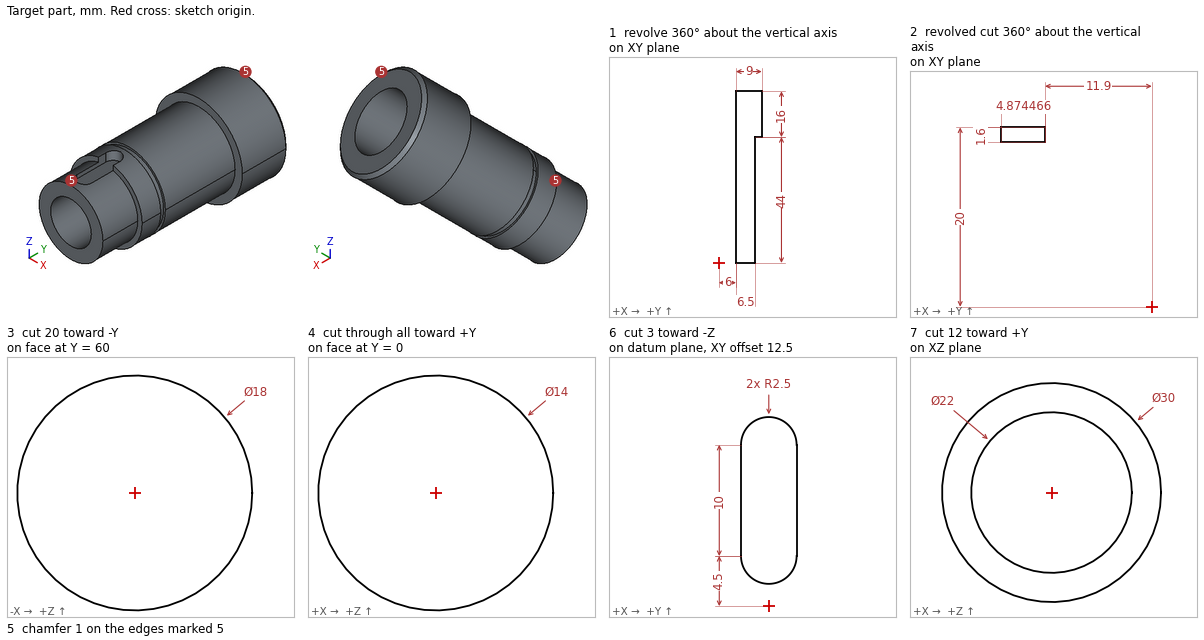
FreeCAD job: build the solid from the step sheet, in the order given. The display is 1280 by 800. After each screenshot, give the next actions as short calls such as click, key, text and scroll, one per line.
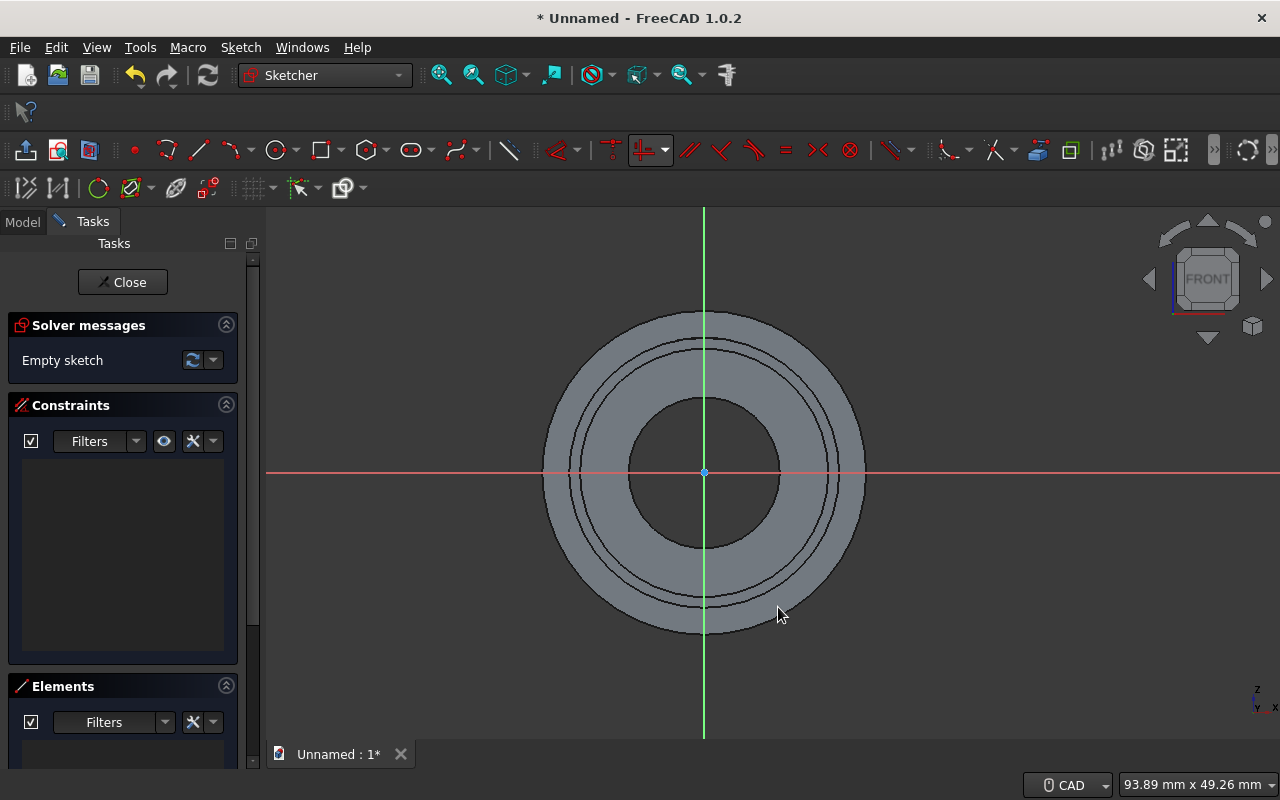
click(276, 150)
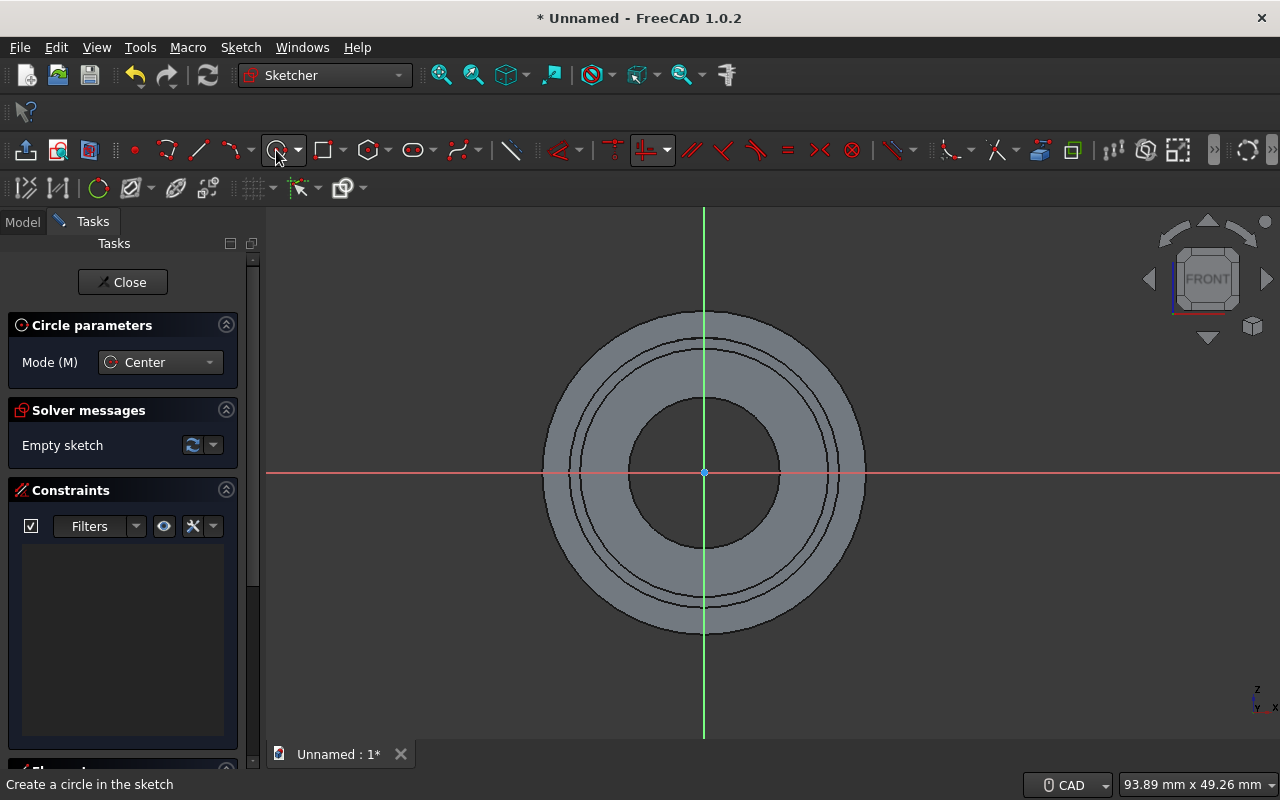
click(704, 473)
move(819, 358)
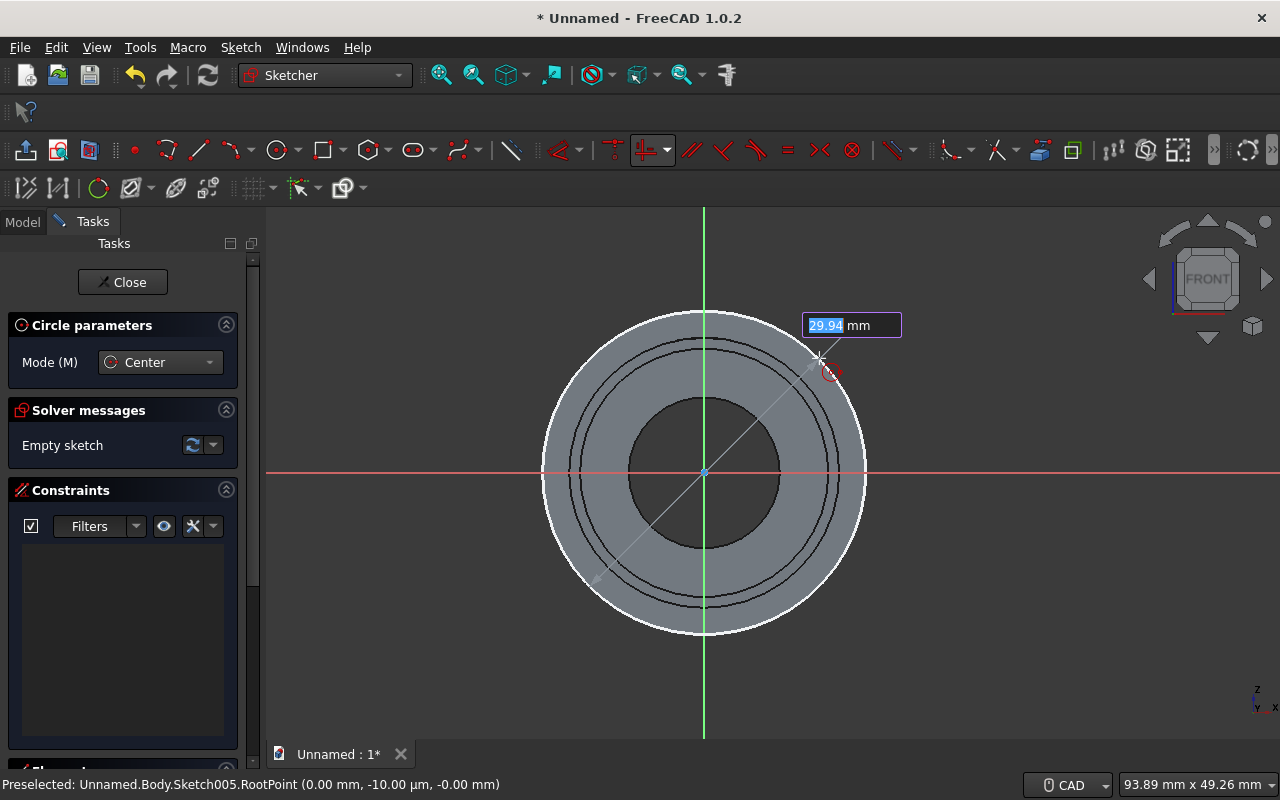
text(30)
key(Return)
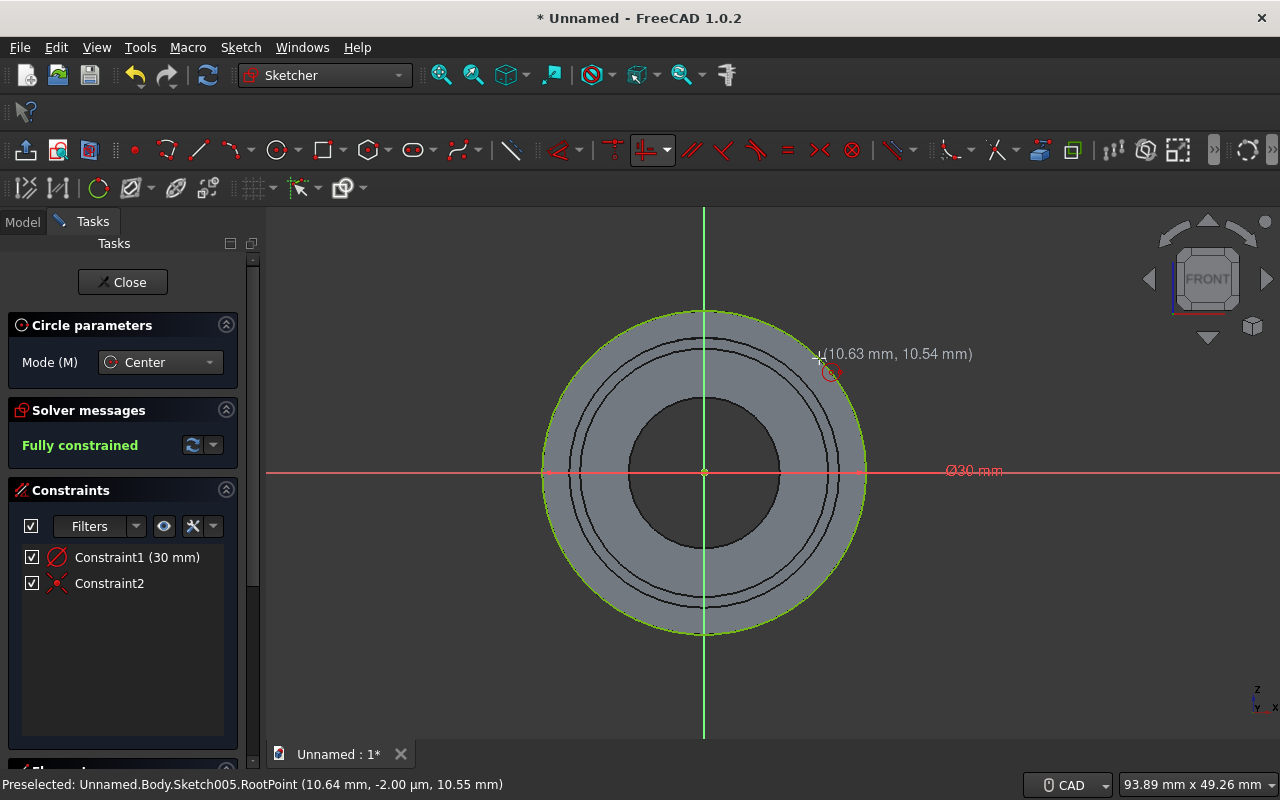
click(704, 473)
move(788, 389)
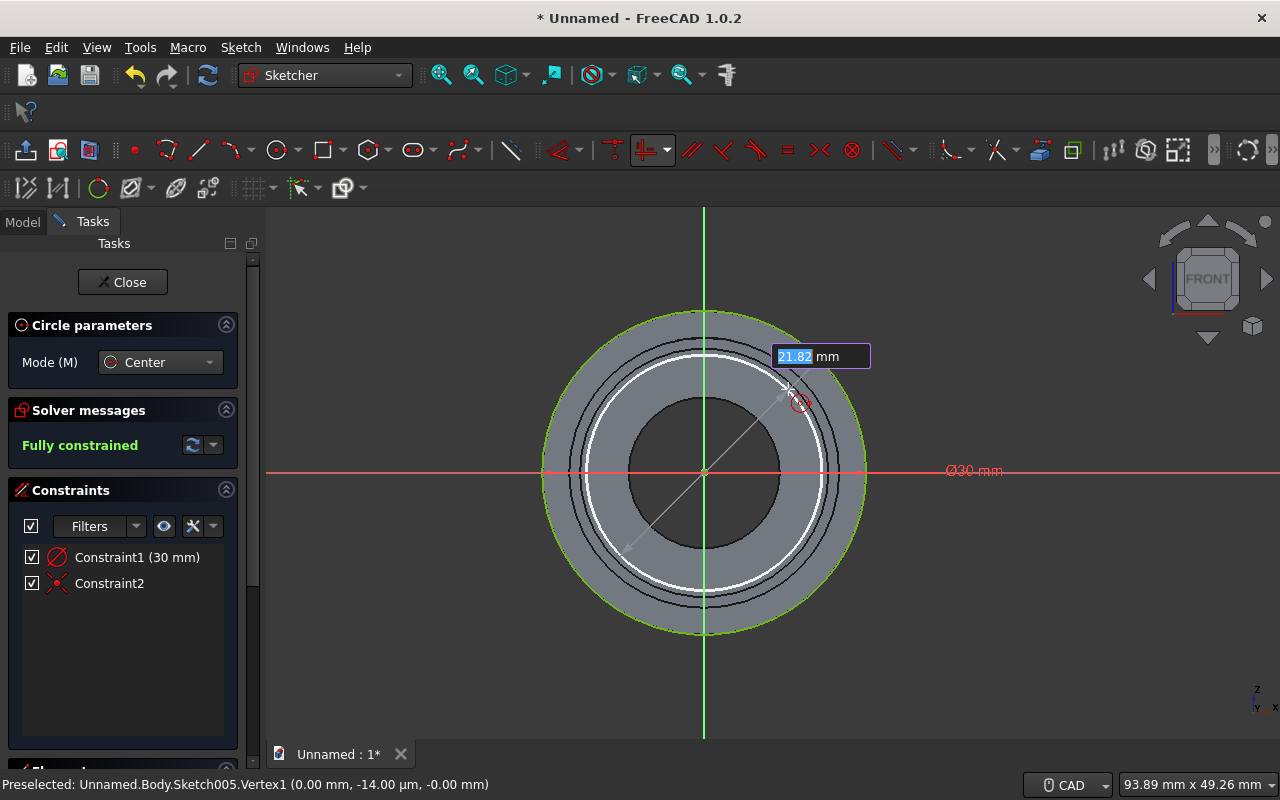
text(22)
key(Return)
key(Escape)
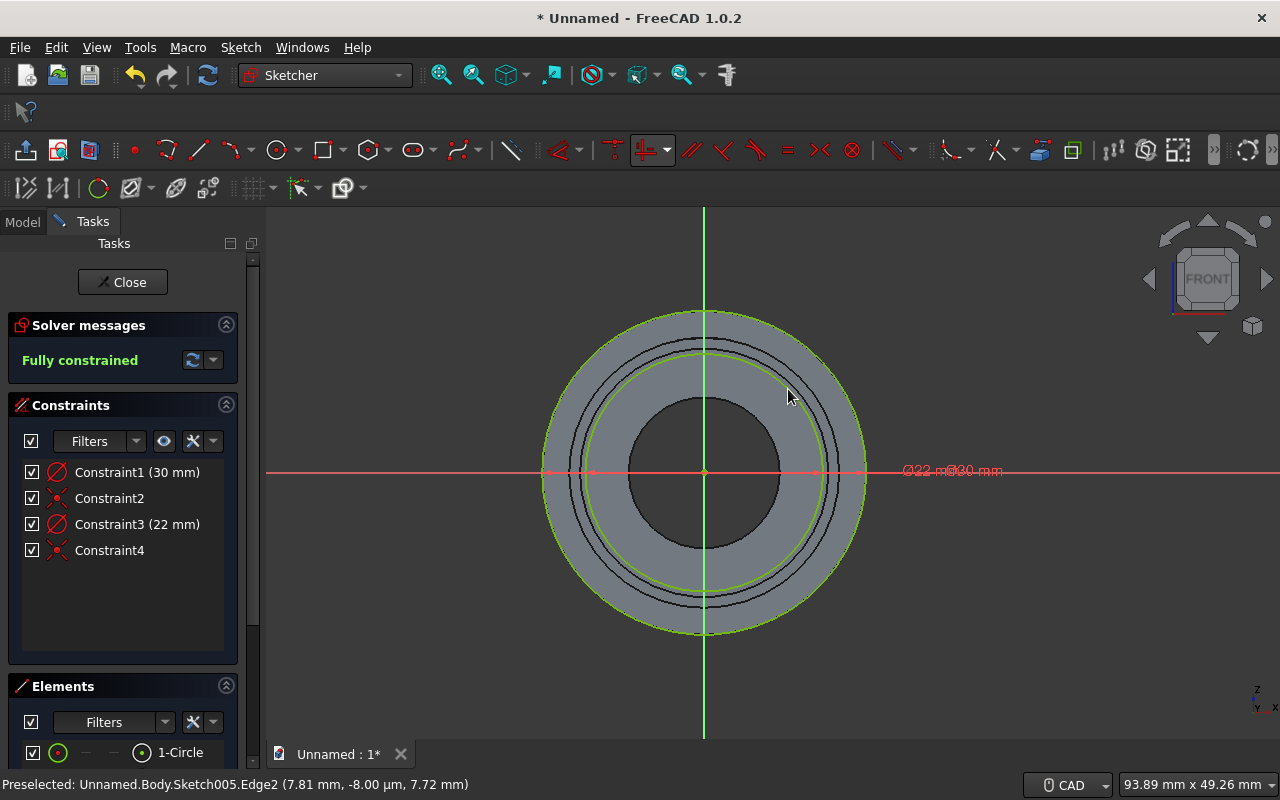
click(123, 282)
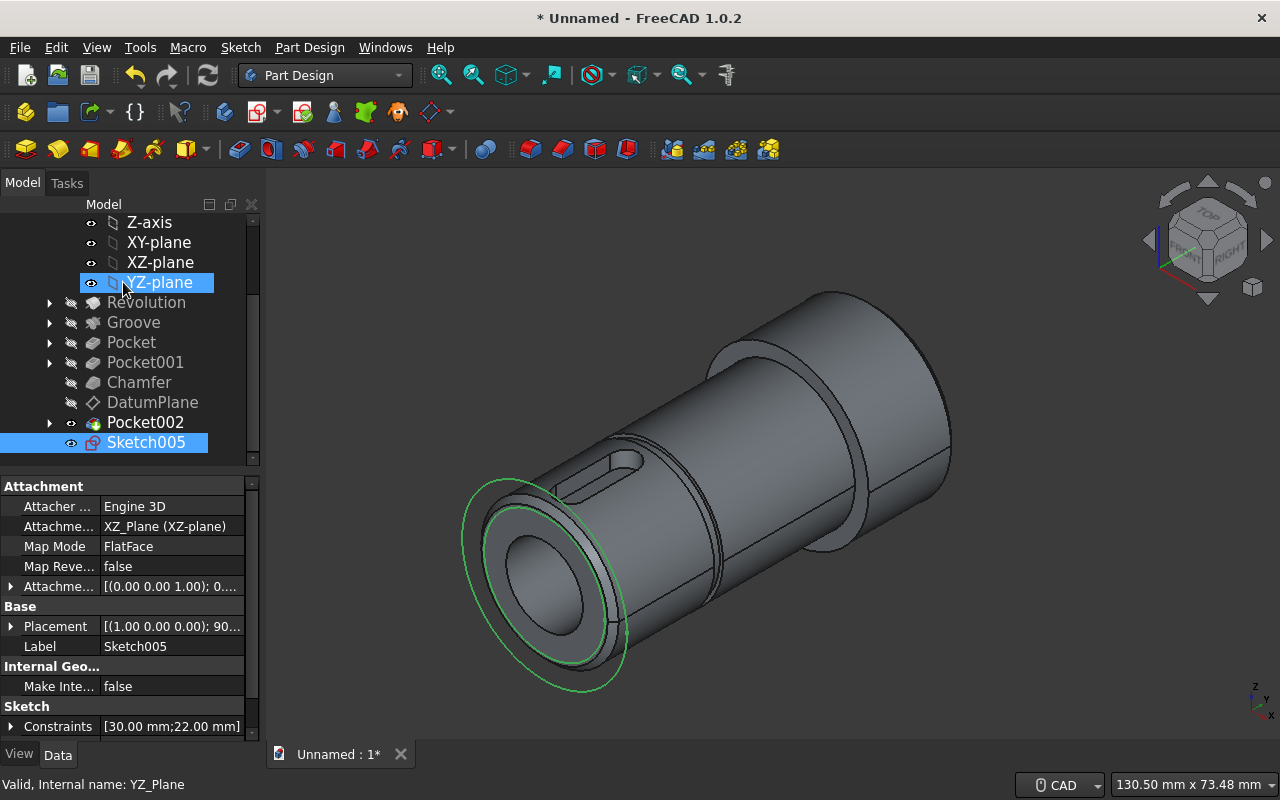
click(240, 150)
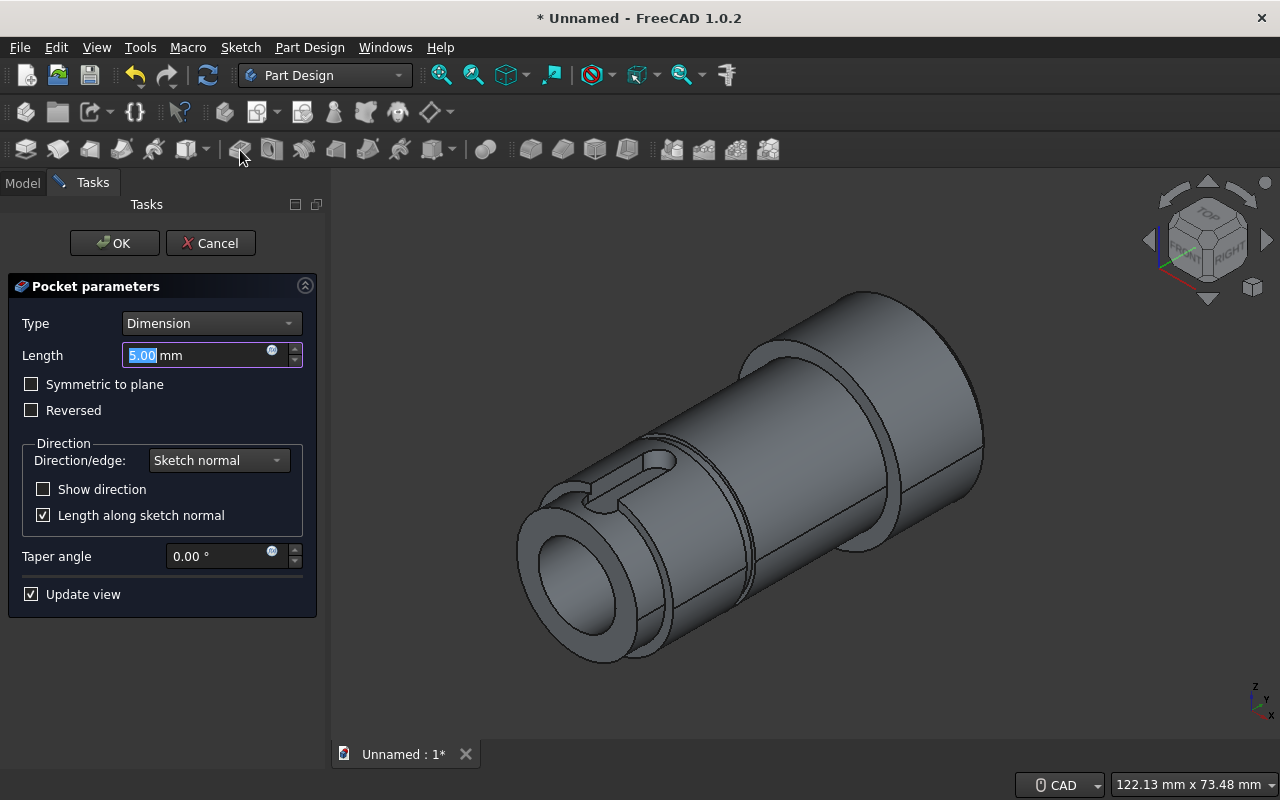
text(12)
key(Tab)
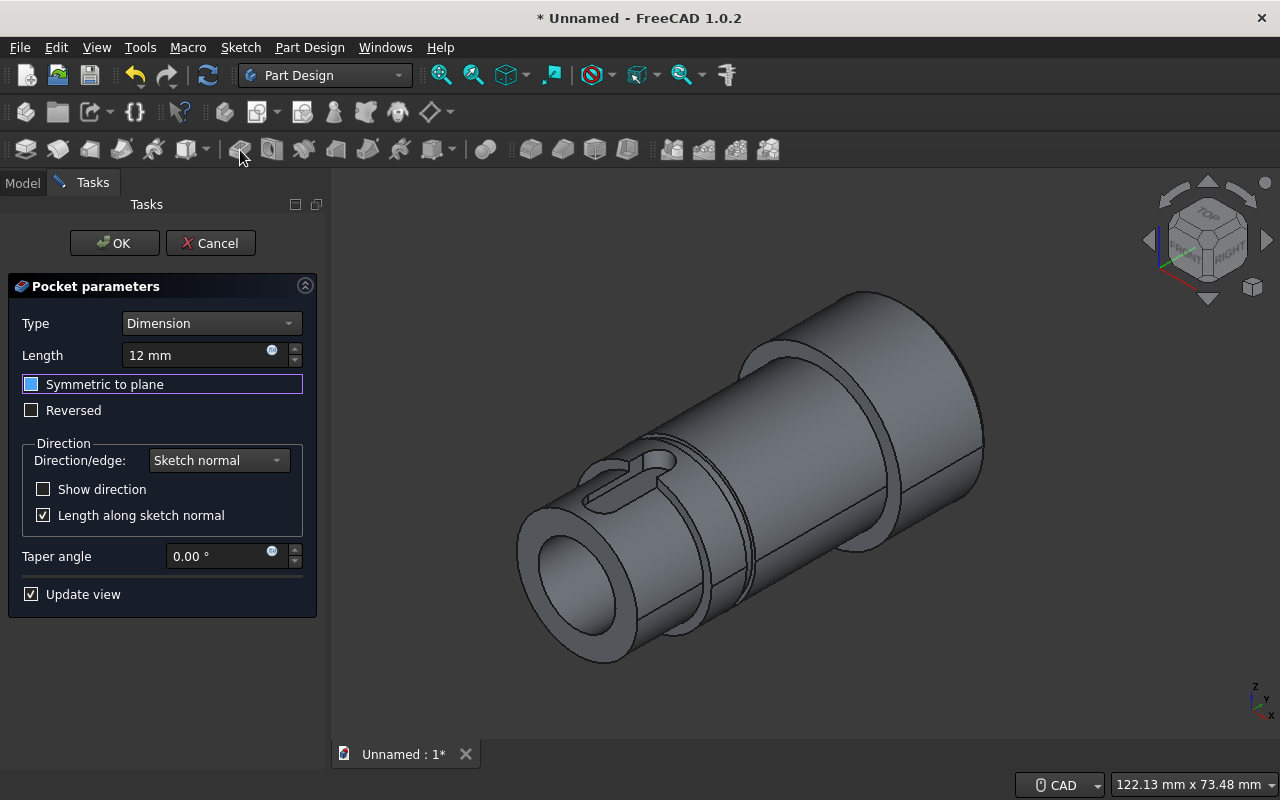
click(115, 243)